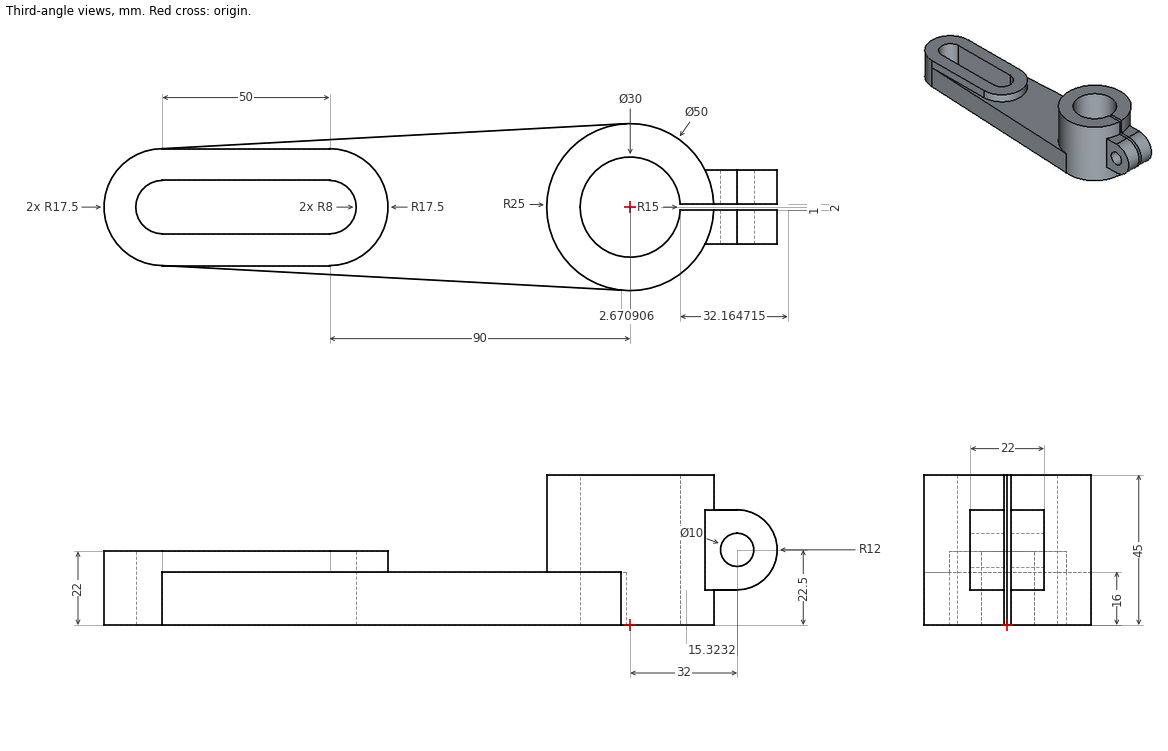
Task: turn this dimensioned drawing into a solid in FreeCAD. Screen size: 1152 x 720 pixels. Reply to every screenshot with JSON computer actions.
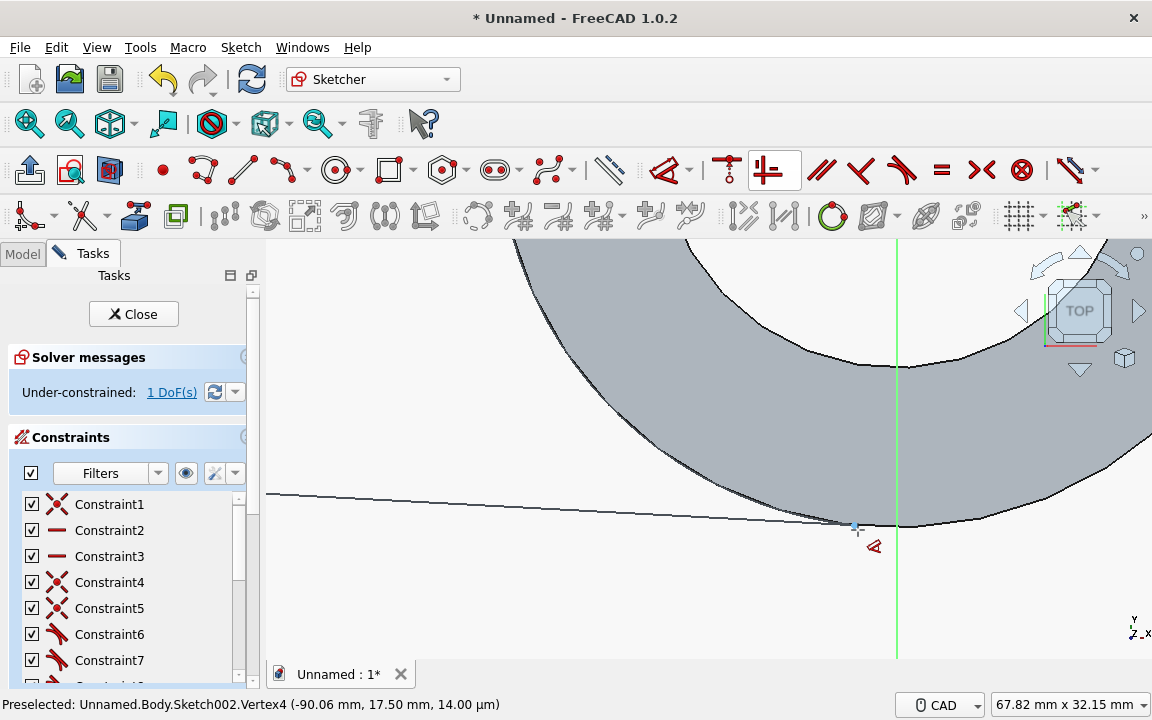
{"action": "left_click", "coordinate": [855, 525]}
{"action": "left_click", "coordinate": [876, 559]}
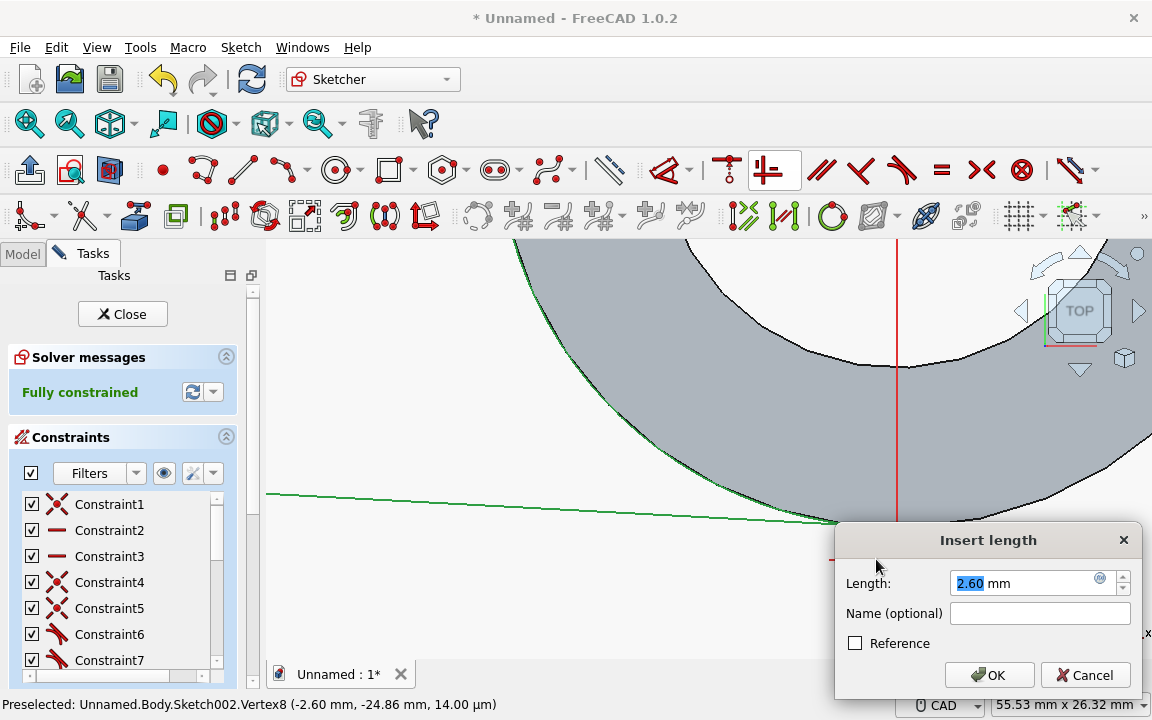
{"action": "type", "text": "2.670906"}
{"action": "key", "text": "Return"}
{"action": "key", "text": "Escape"}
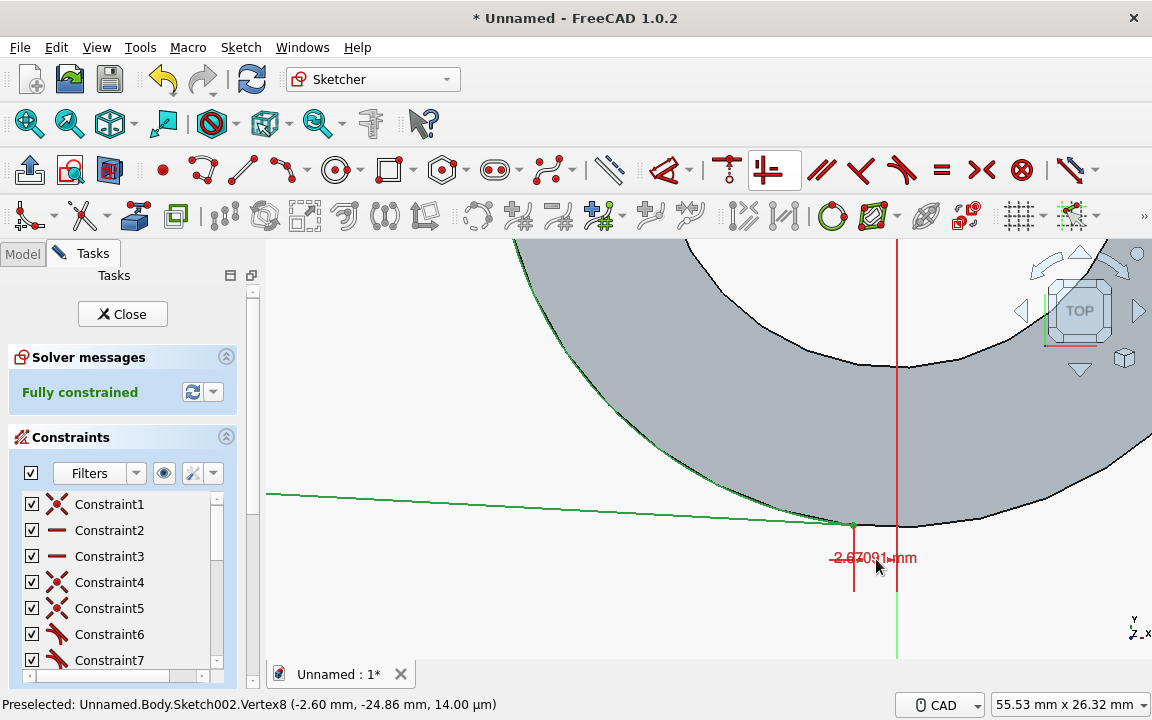
{"action": "left_click", "coordinate": [123, 314]}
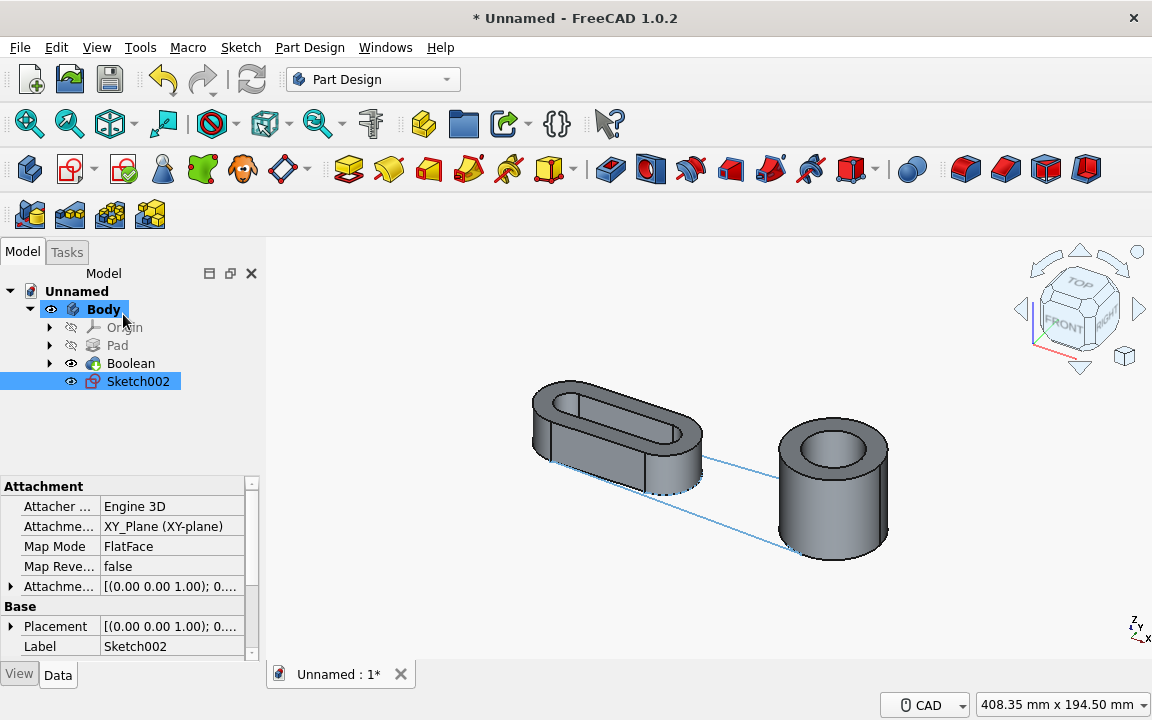
{"action": "left_click", "coordinate": [350, 170]}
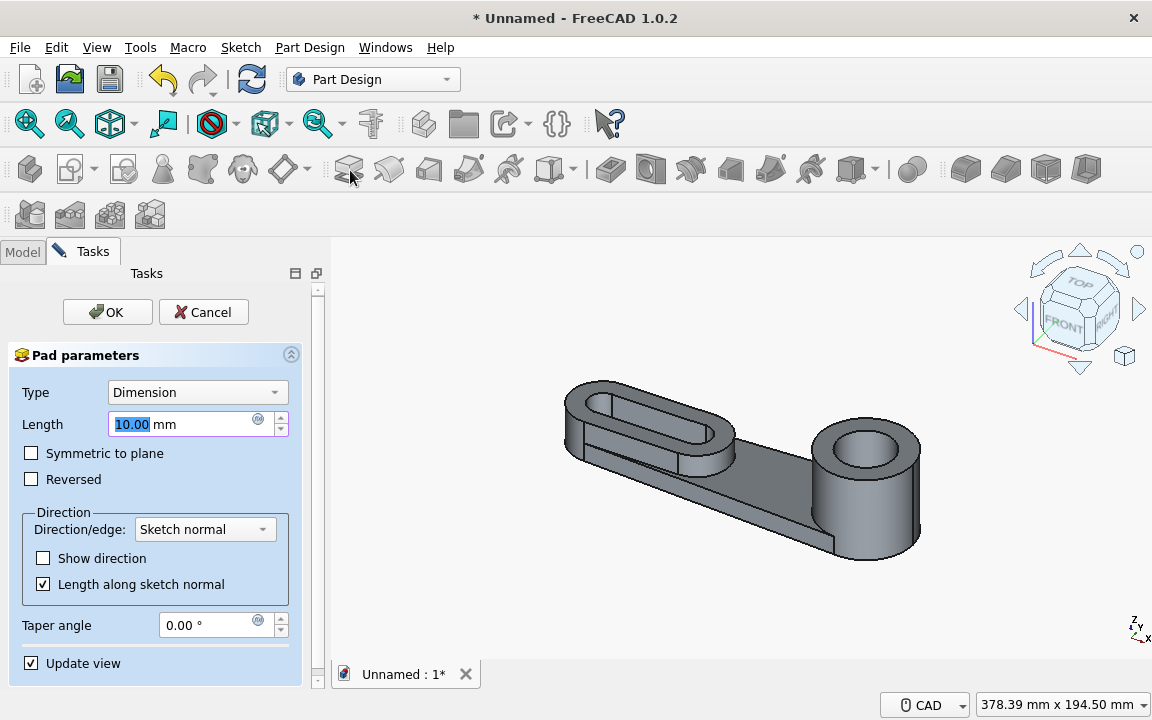
{"action": "type", "text": "16"}
{"action": "key", "text": "Tab"}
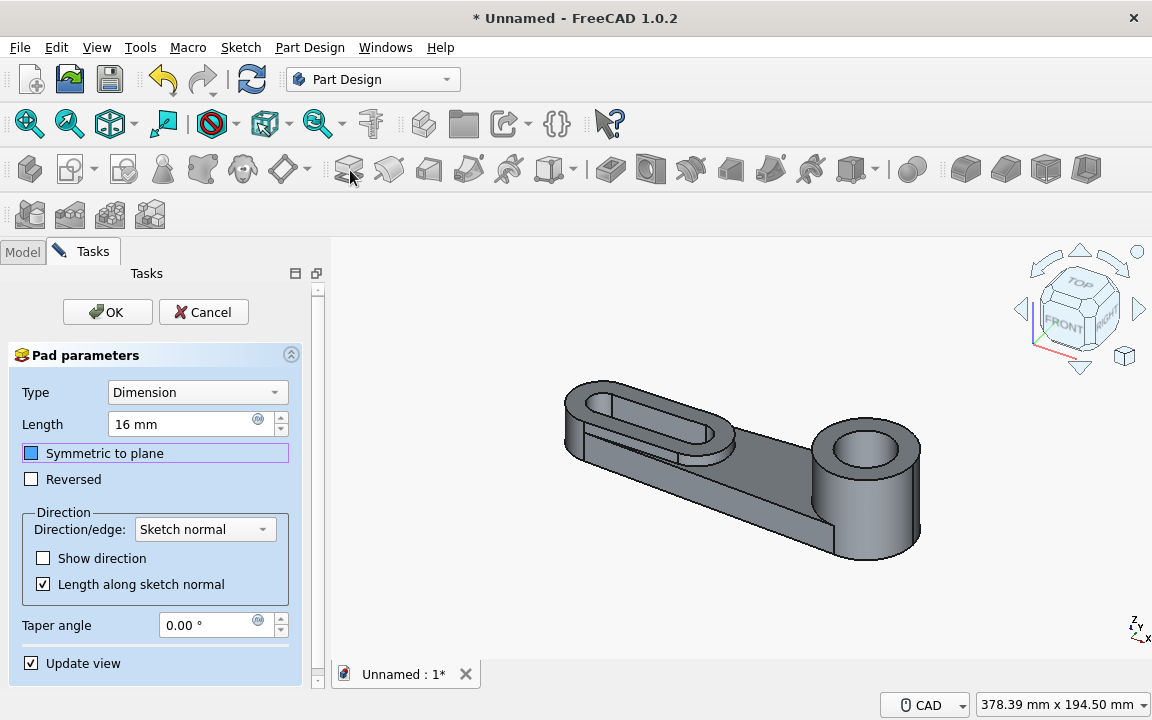
{"action": "left_click", "coordinate": [108, 312]}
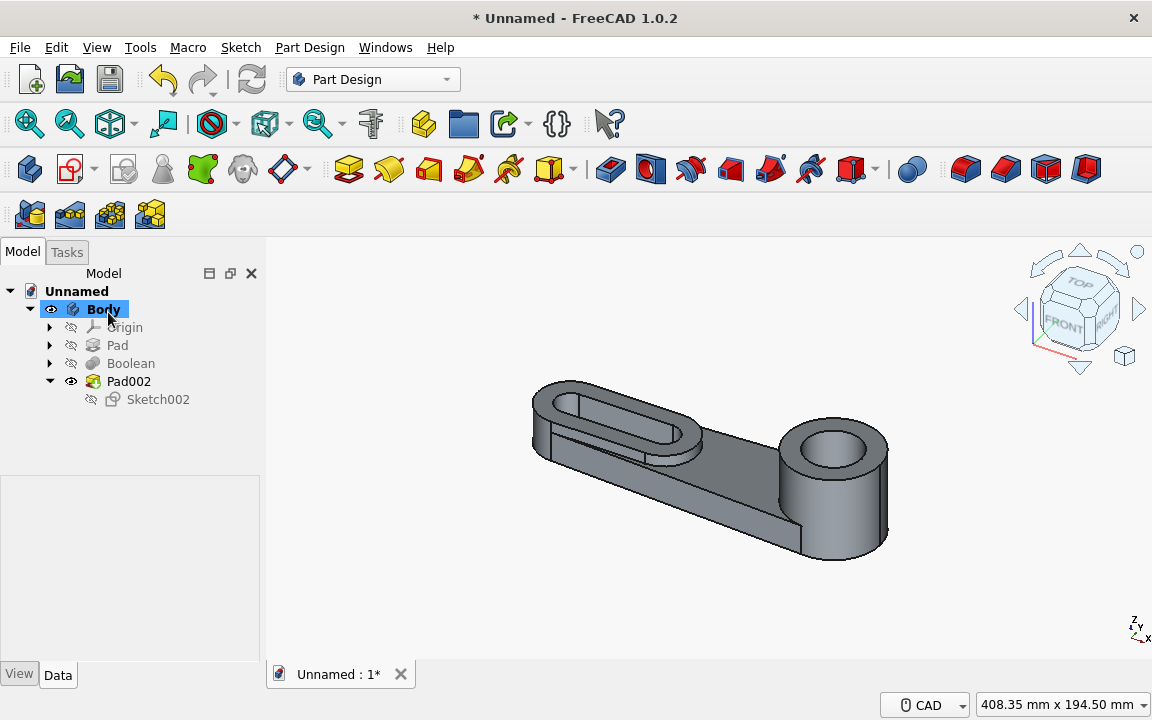
{"action": "left_click", "coordinate": [70, 170]}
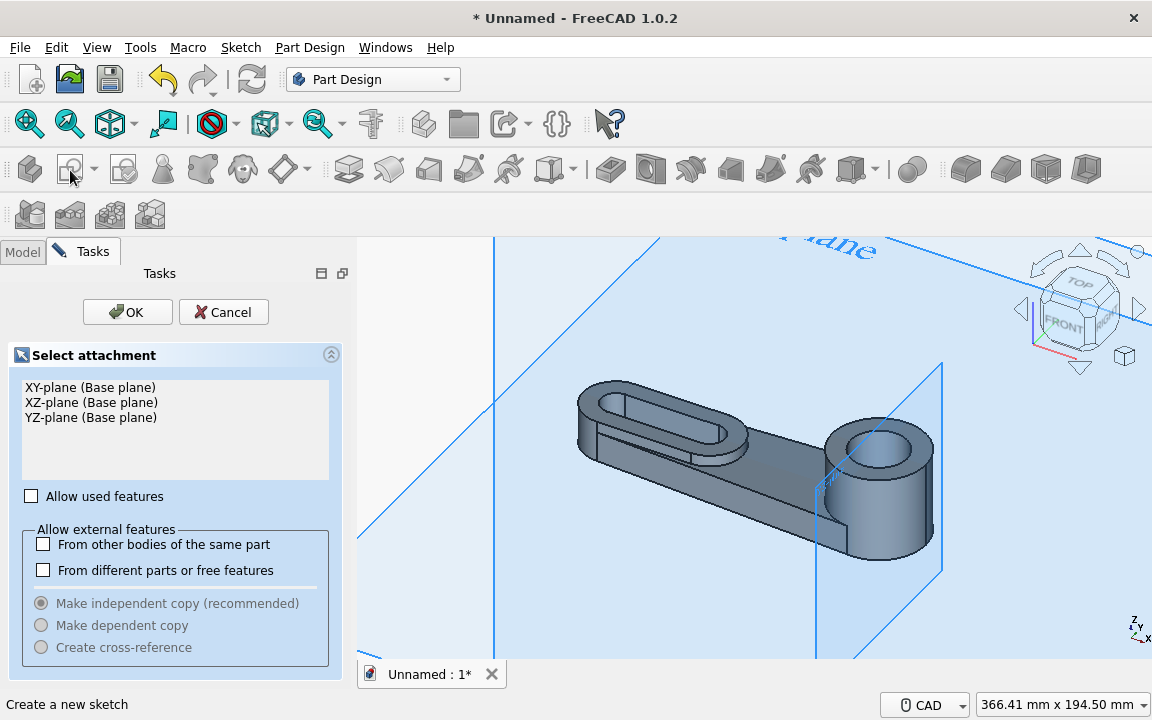
{"action": "left_click", "coordinate": [82, 402]}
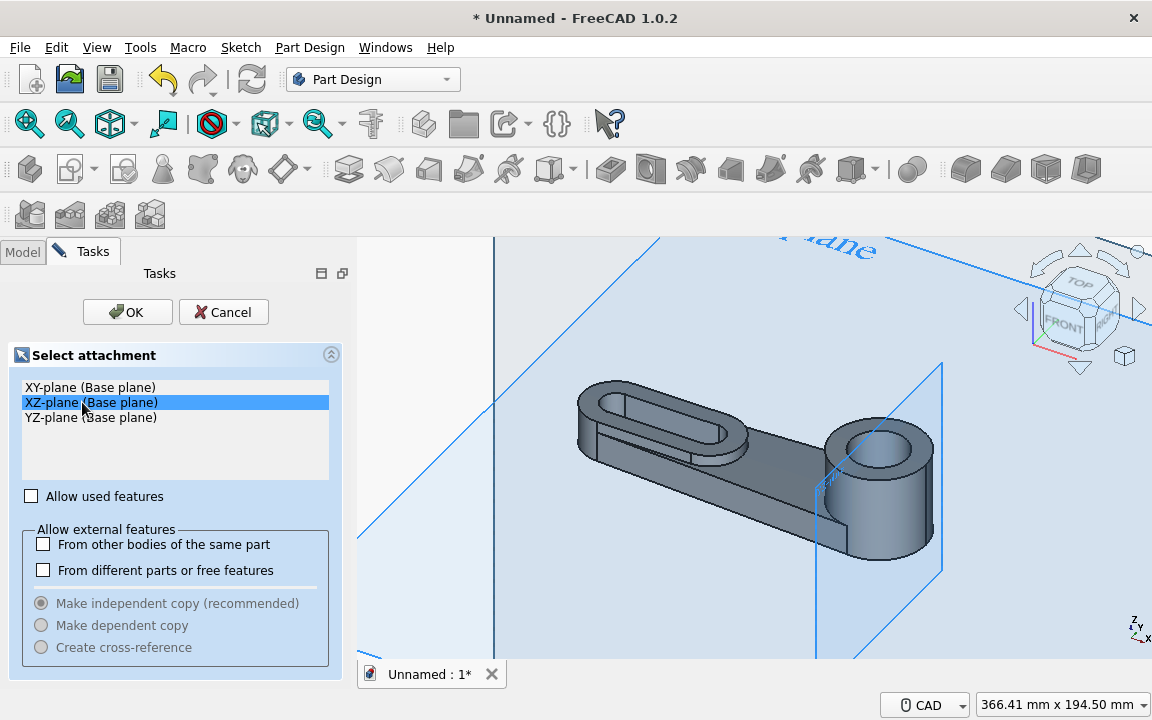
{"action": "left_click", "coordinate": [128, 312]}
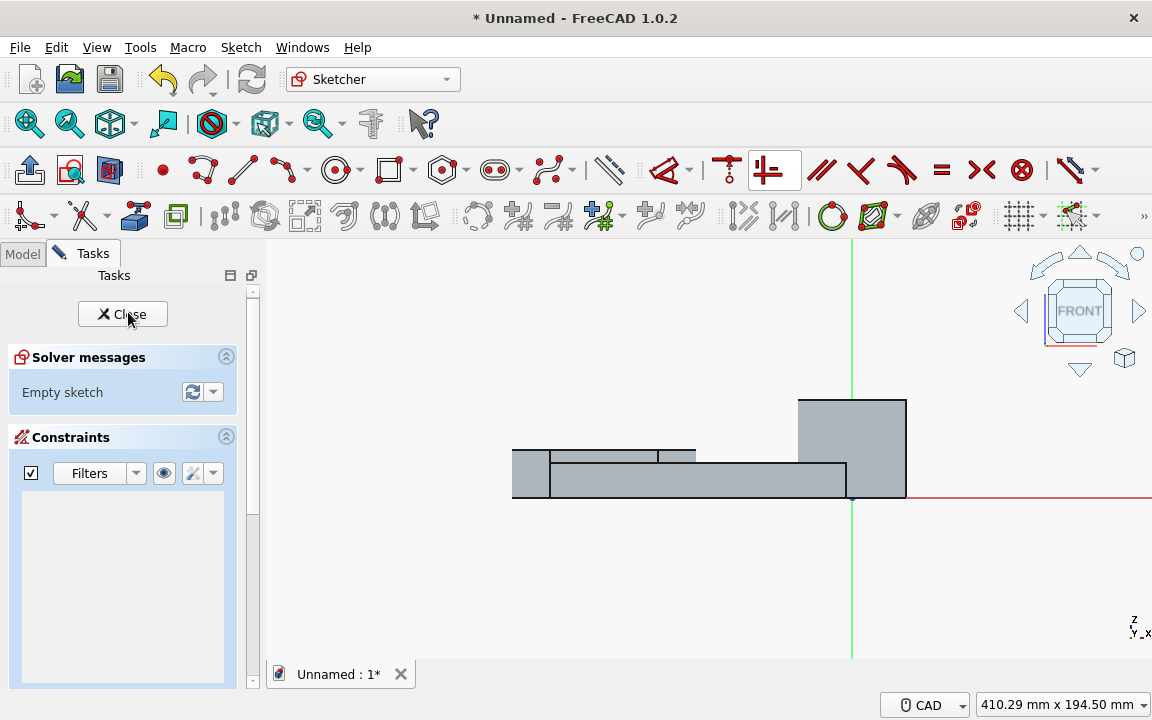
{"action": "left_click", "coordinate": [110, 170]}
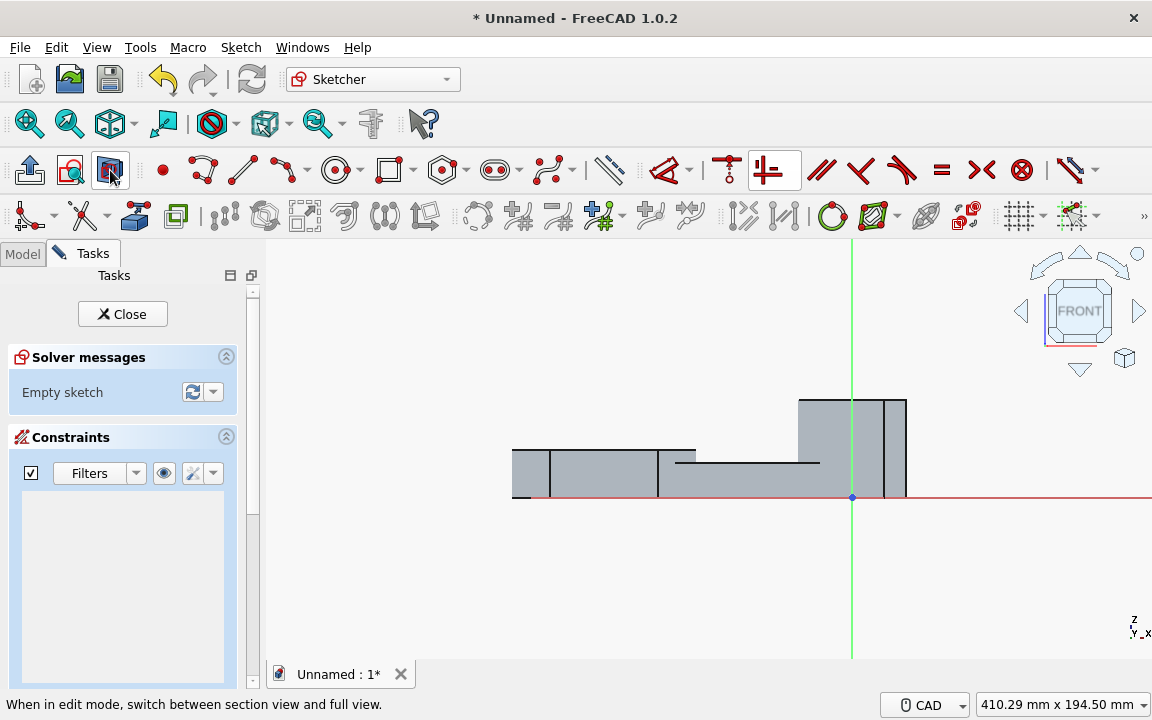
{"action": "scroll", "coordinate": [987, 465], "scroll_direction": "up", "scroll_amount": 6}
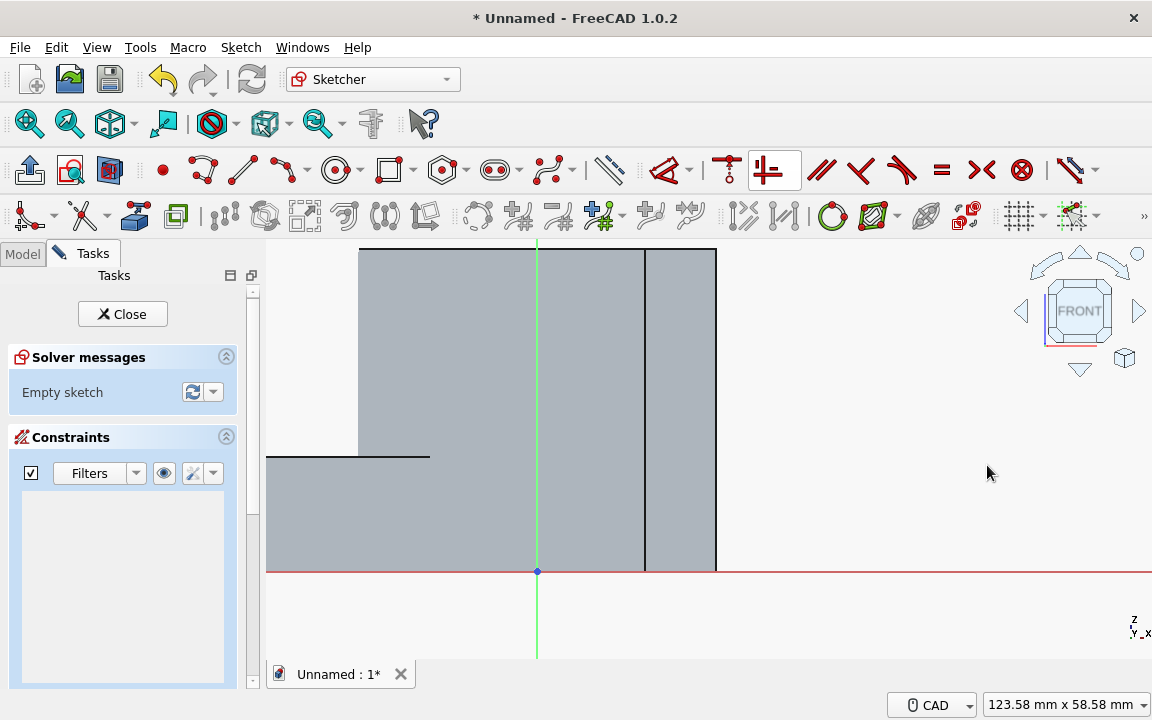
{"action": "left_click", "coordinate": [204, 170]}